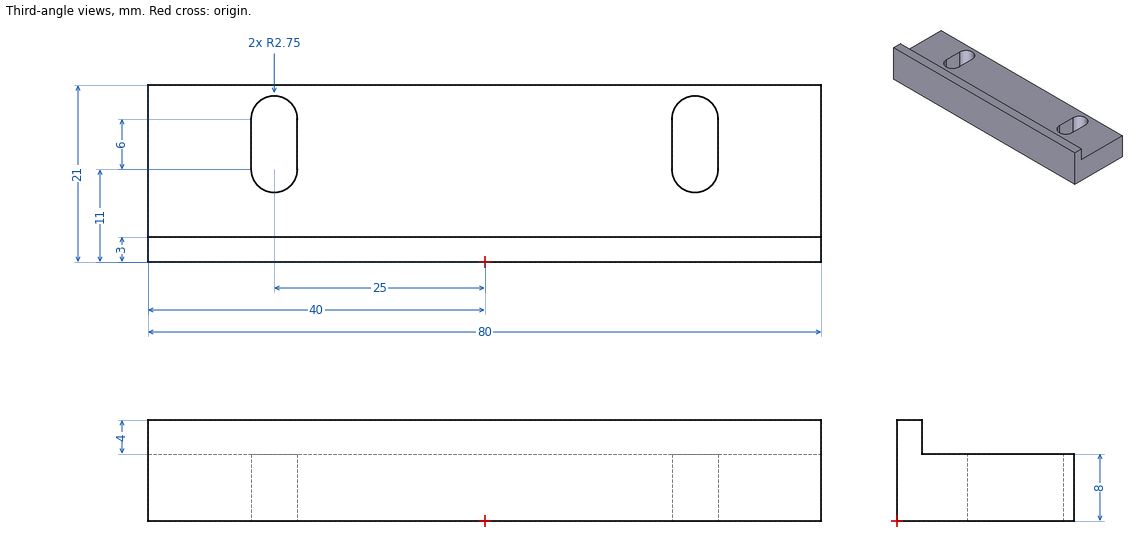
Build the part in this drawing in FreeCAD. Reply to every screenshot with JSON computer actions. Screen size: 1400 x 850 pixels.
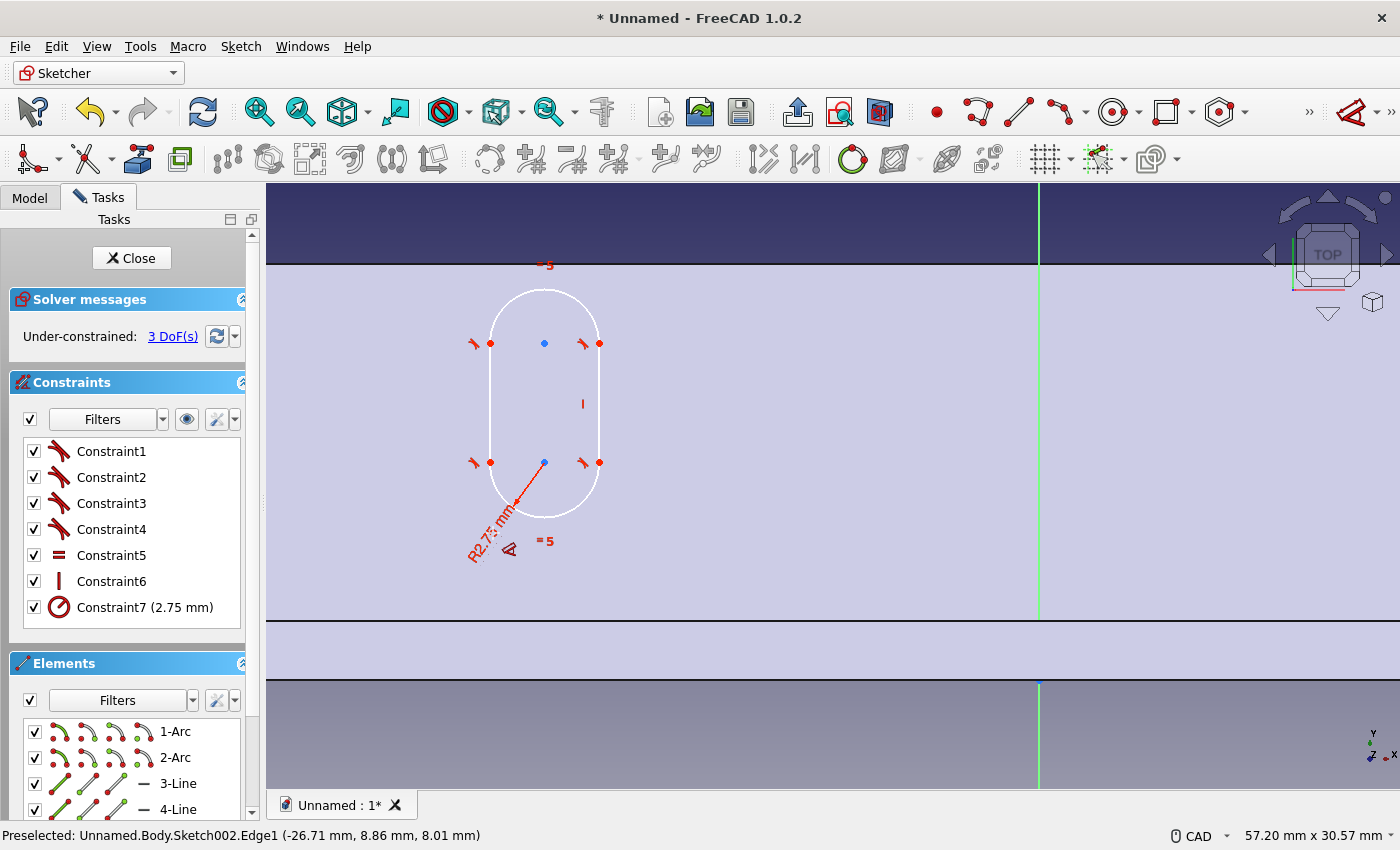
{"action": "left_click", "coordinate": [490, 427]}
{"action": "left_click", "coordinate": [456, 404]}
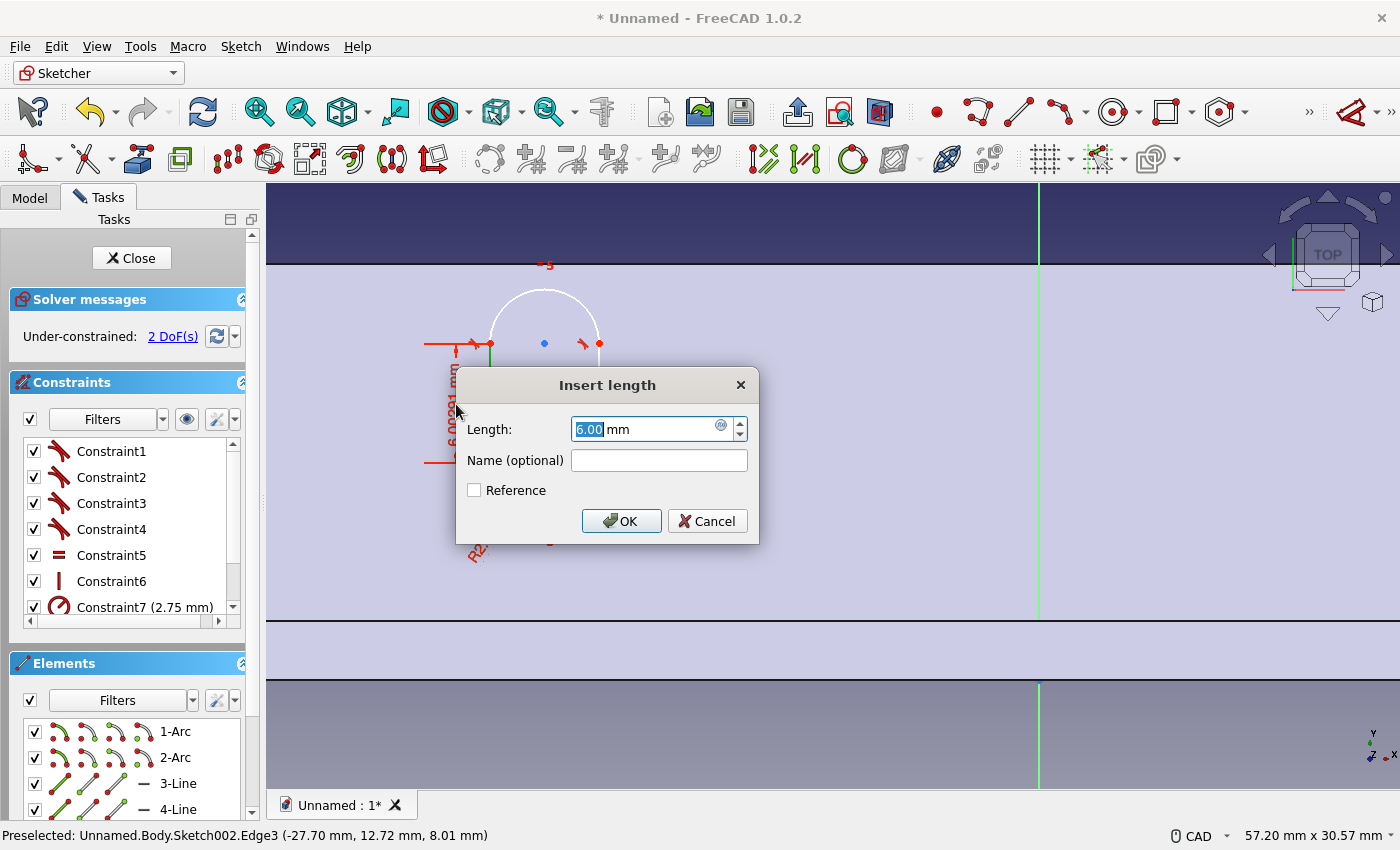
{"action": "type", "text": "6"}
{"action": "key", "text": "Return"}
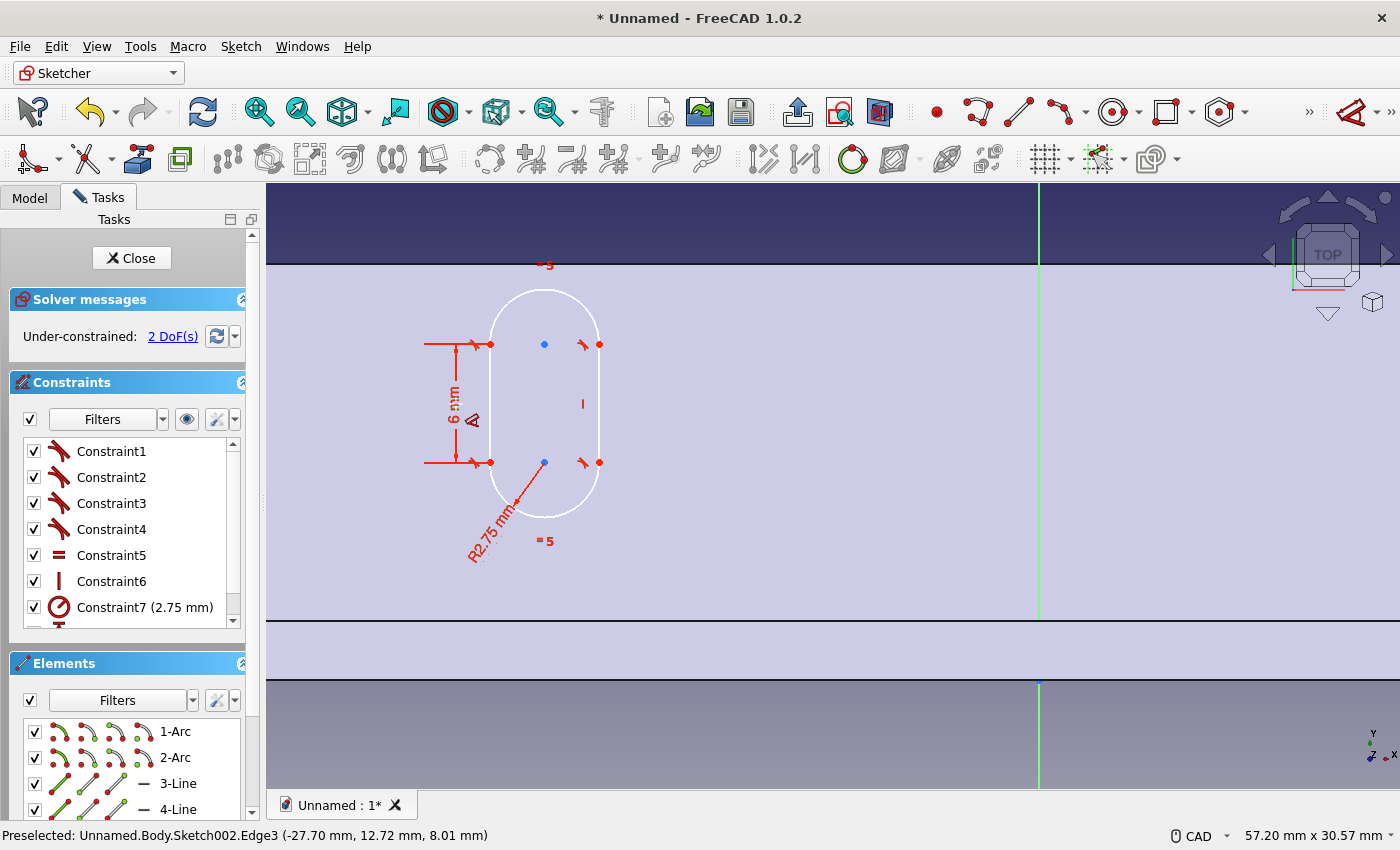
{"action": "left_click", "coordinate": [490, 463]}
{"action": "left_click", "coordinate": [1073, 572]}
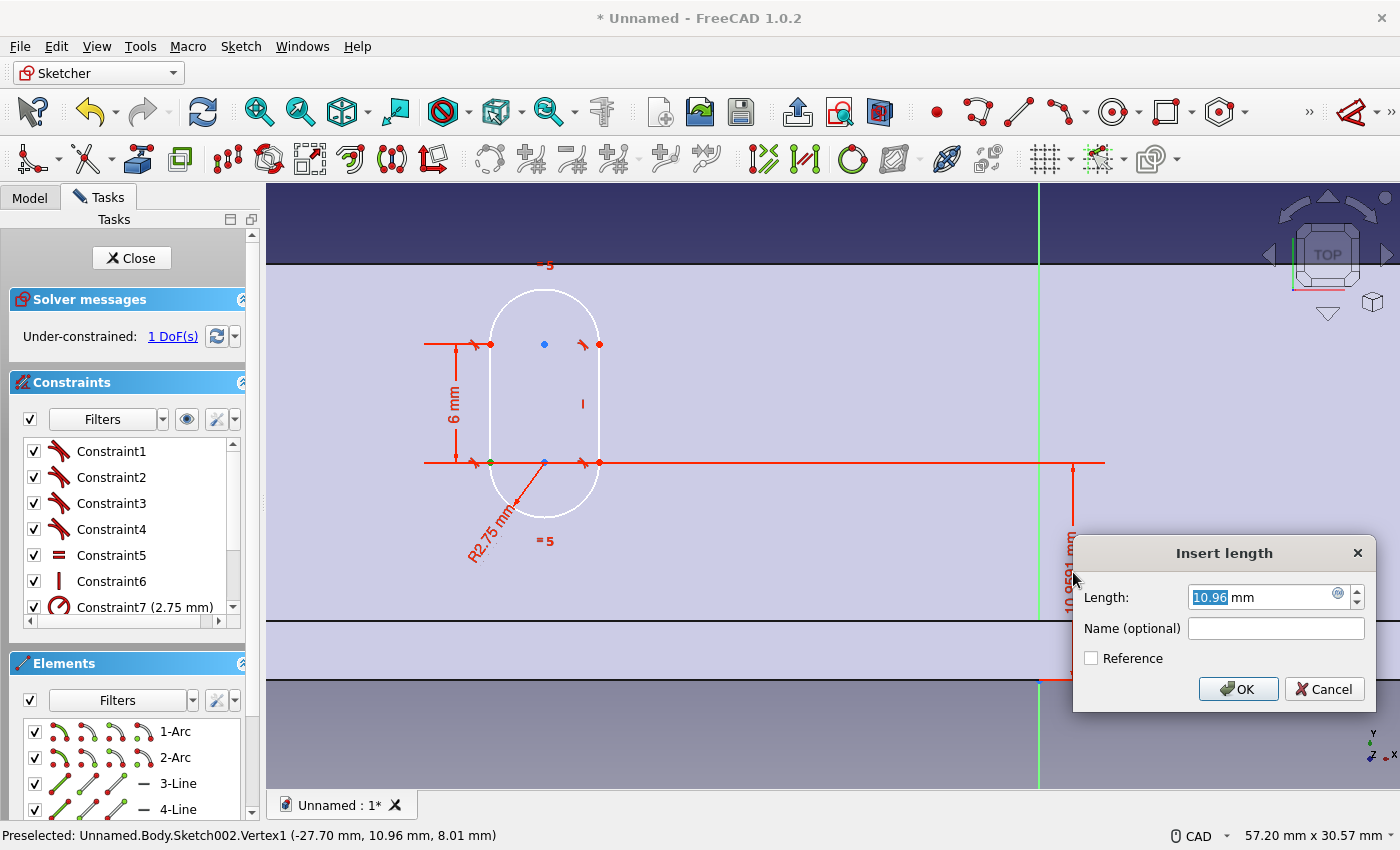
{"action": "type", "text": "11"}
{"action": "key", "text": "Return"}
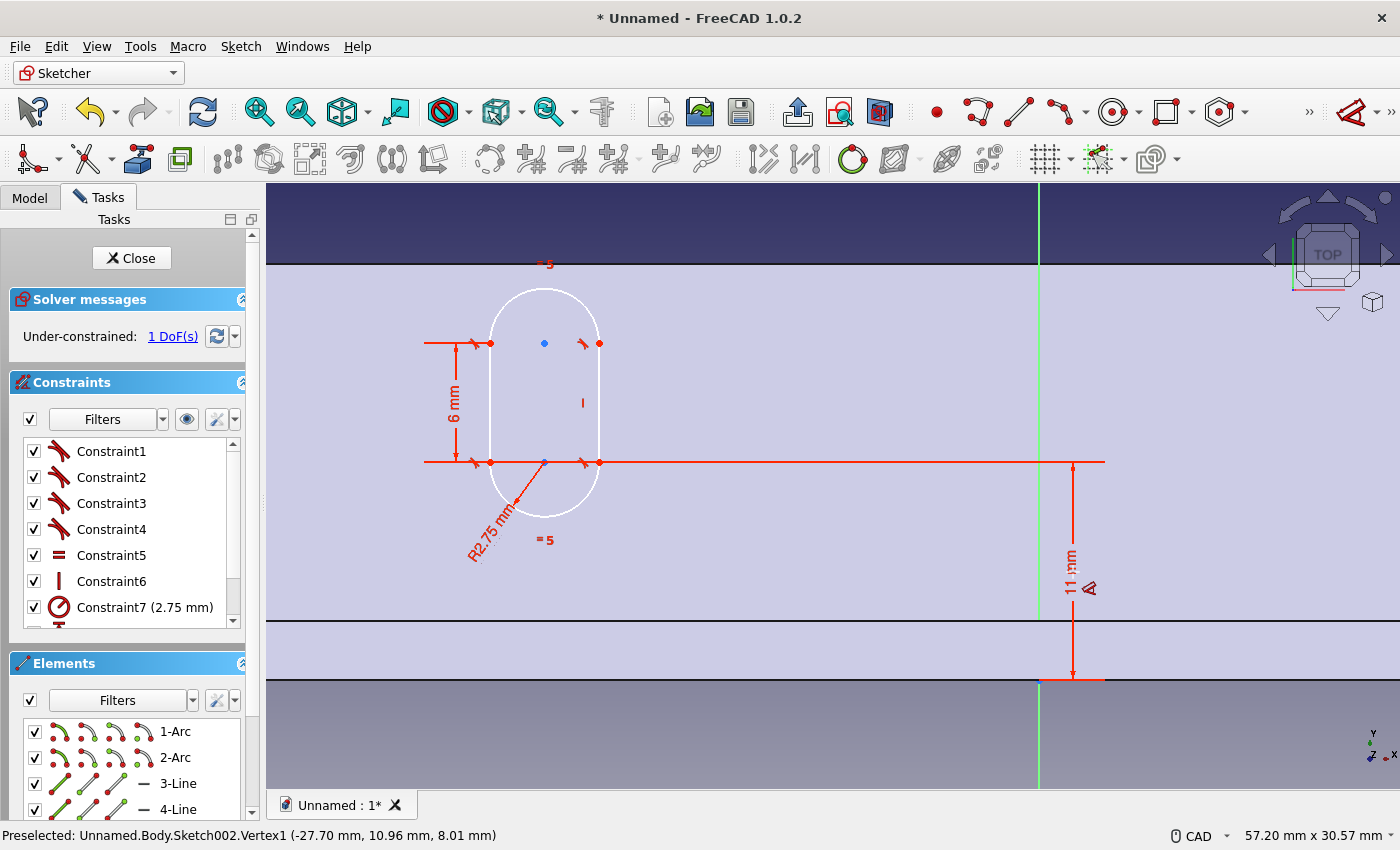
{"action": "left_click", "coordinate": [545, 462]}
{"action": "left_click", "coordinate": [792, 714]}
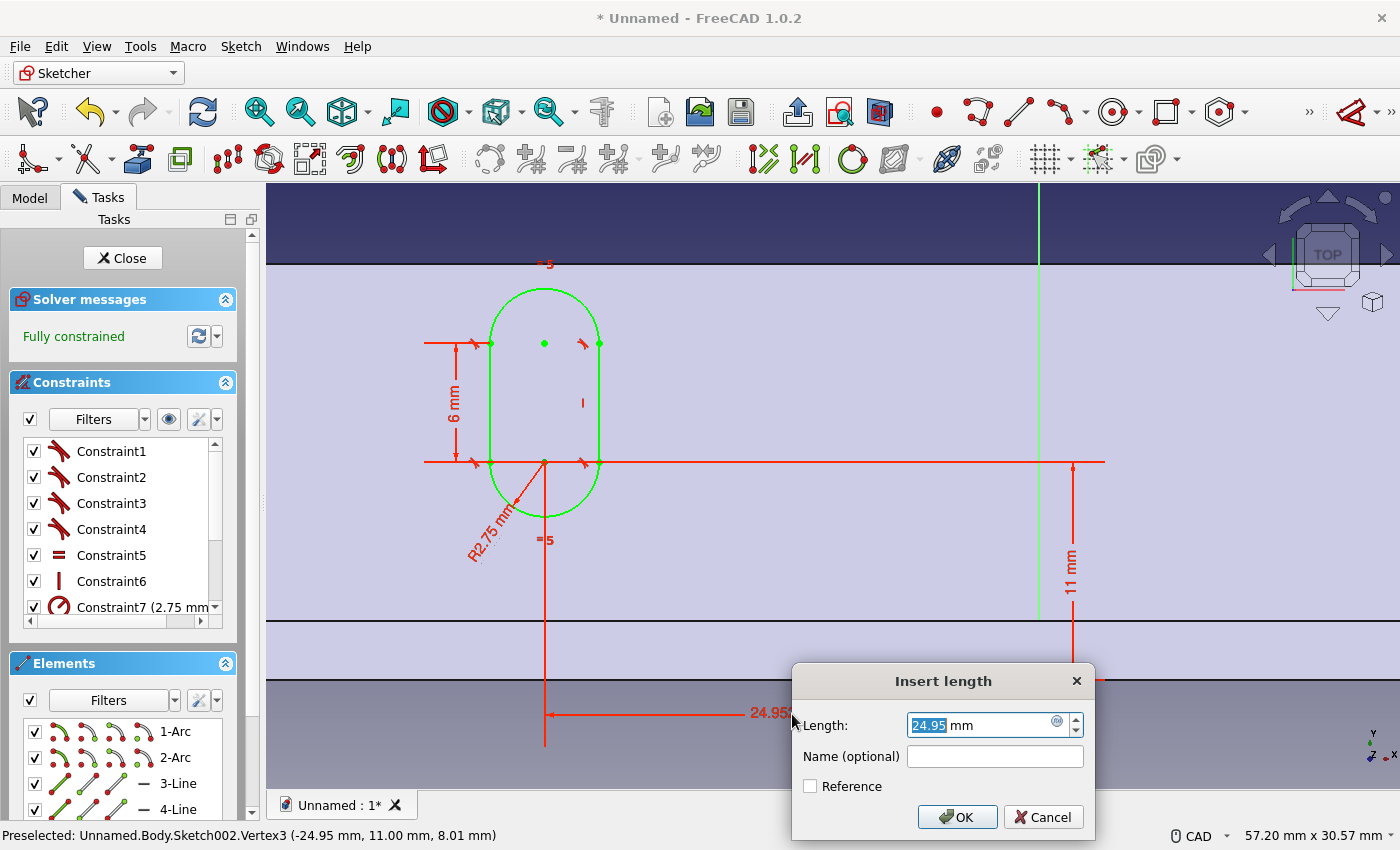
{"action": "type", "text": "25"}
{"action": "key", "text": "Return"}
{"action": "key", "text": "Escape"}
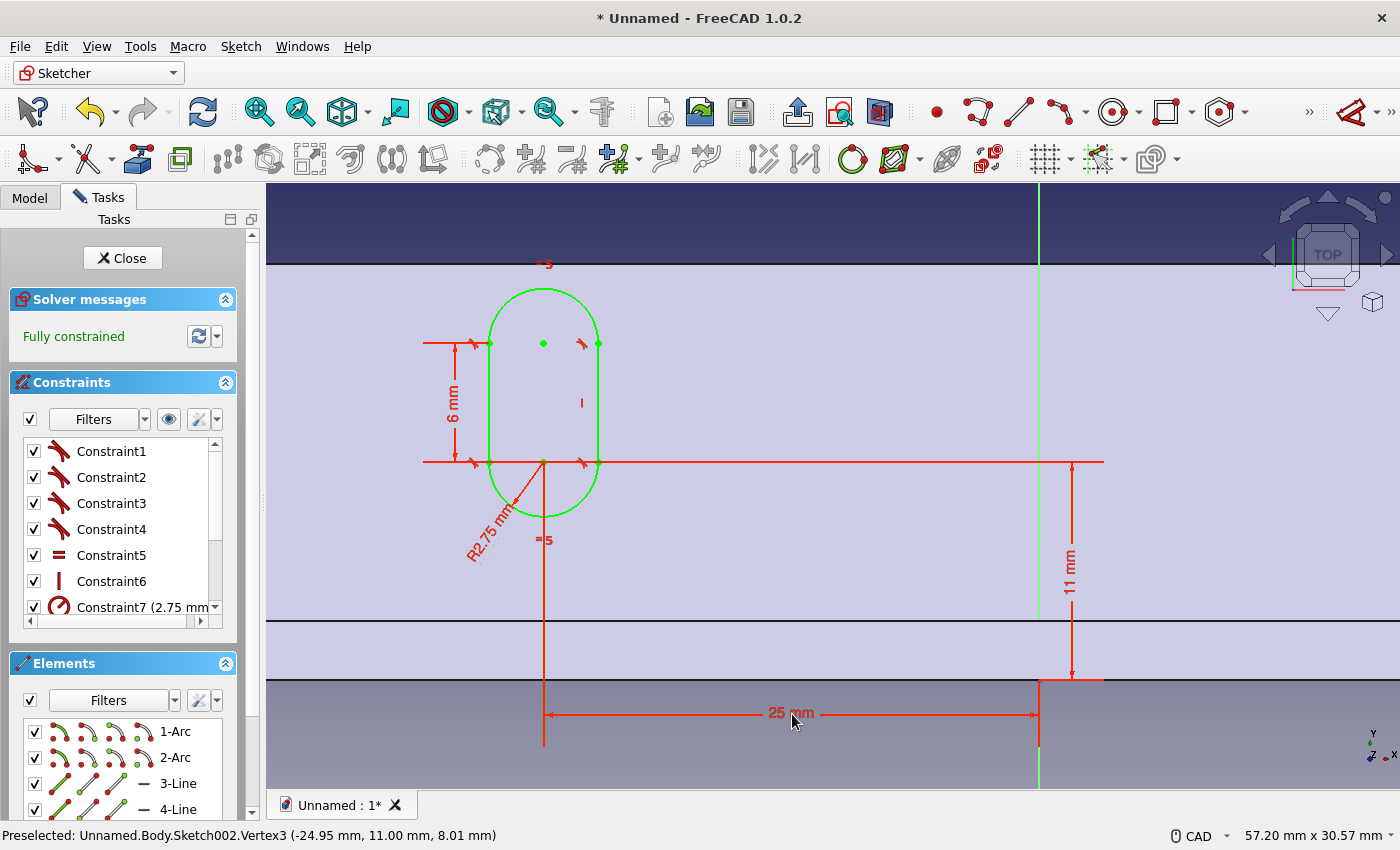
{"action": "left_click", "coordinate": [123, 258]}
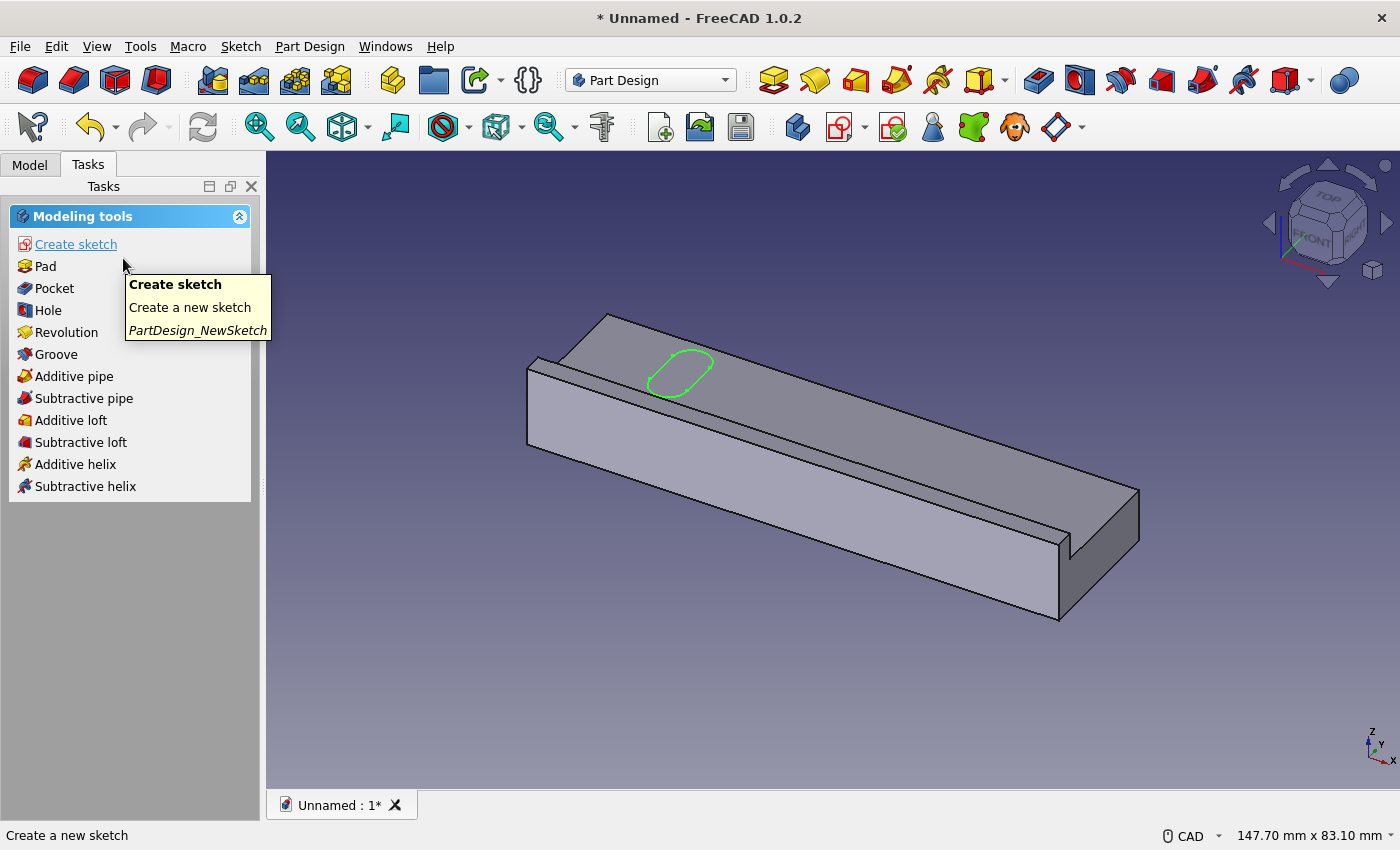
{"action": "left_click", "coordinate": [1039, 80]}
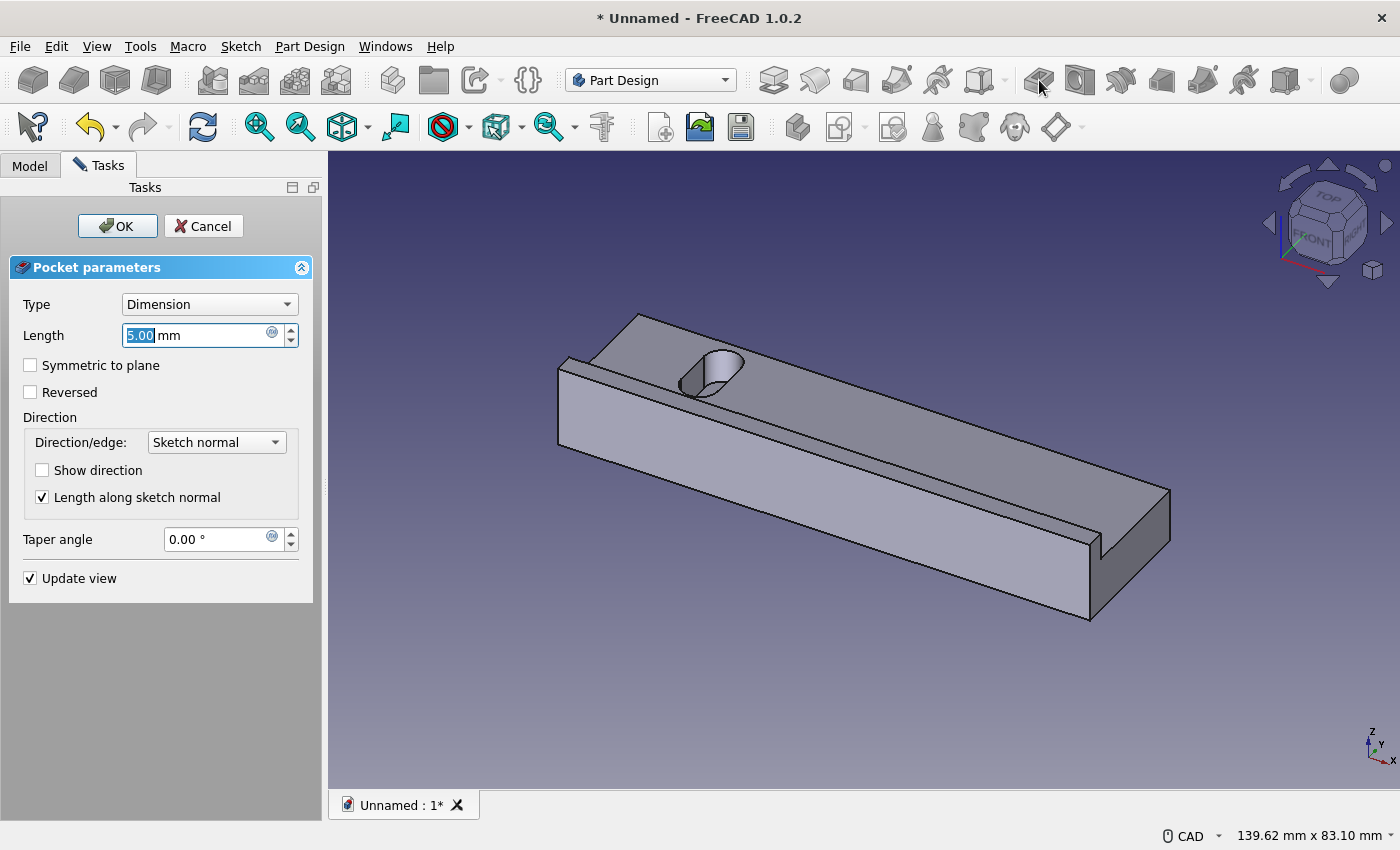
{"action": "type", "text": "8"}
{"action": "key", "text": "Tab"}